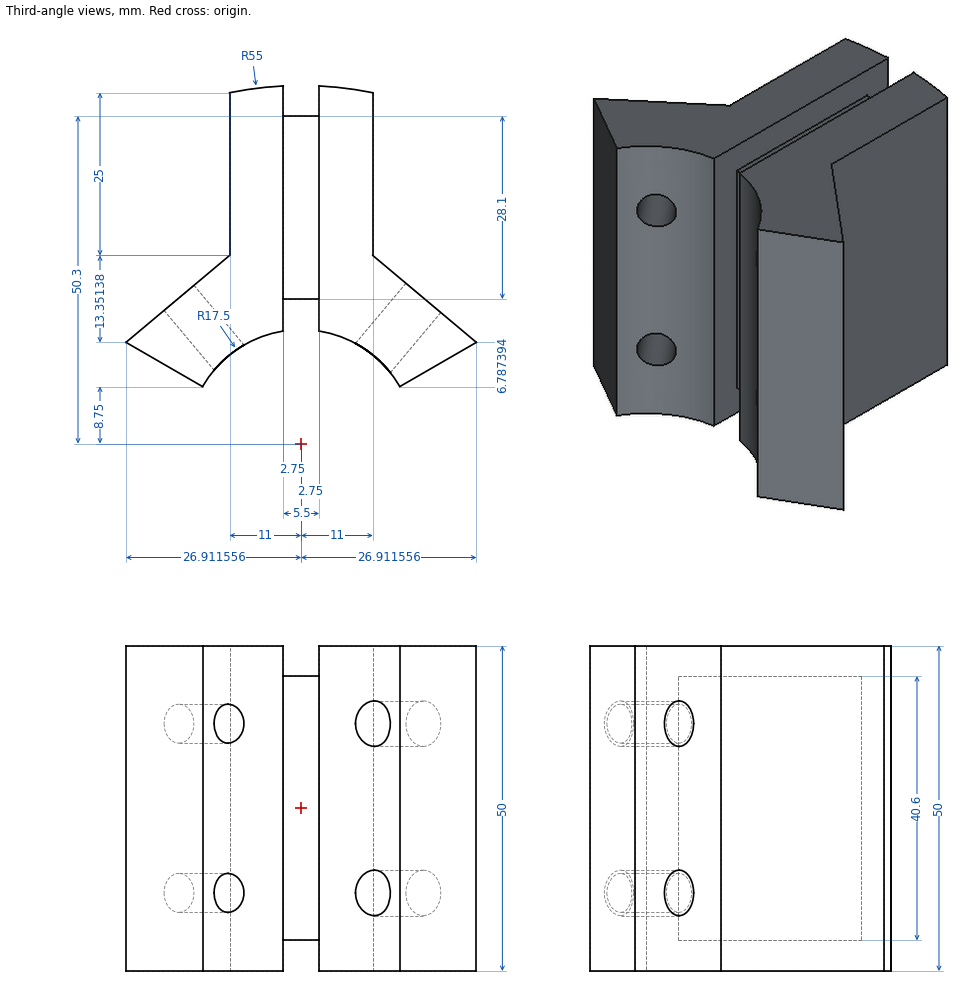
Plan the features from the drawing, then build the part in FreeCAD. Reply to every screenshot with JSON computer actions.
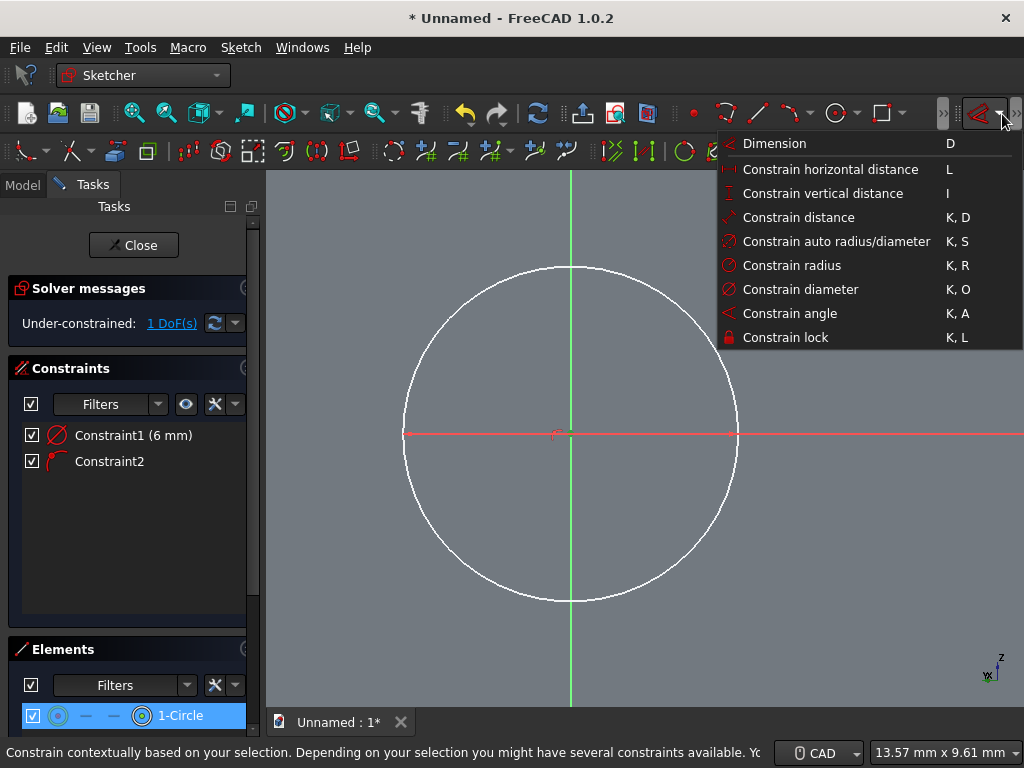
{"action": "left_click", "coordinate": [870, 193]}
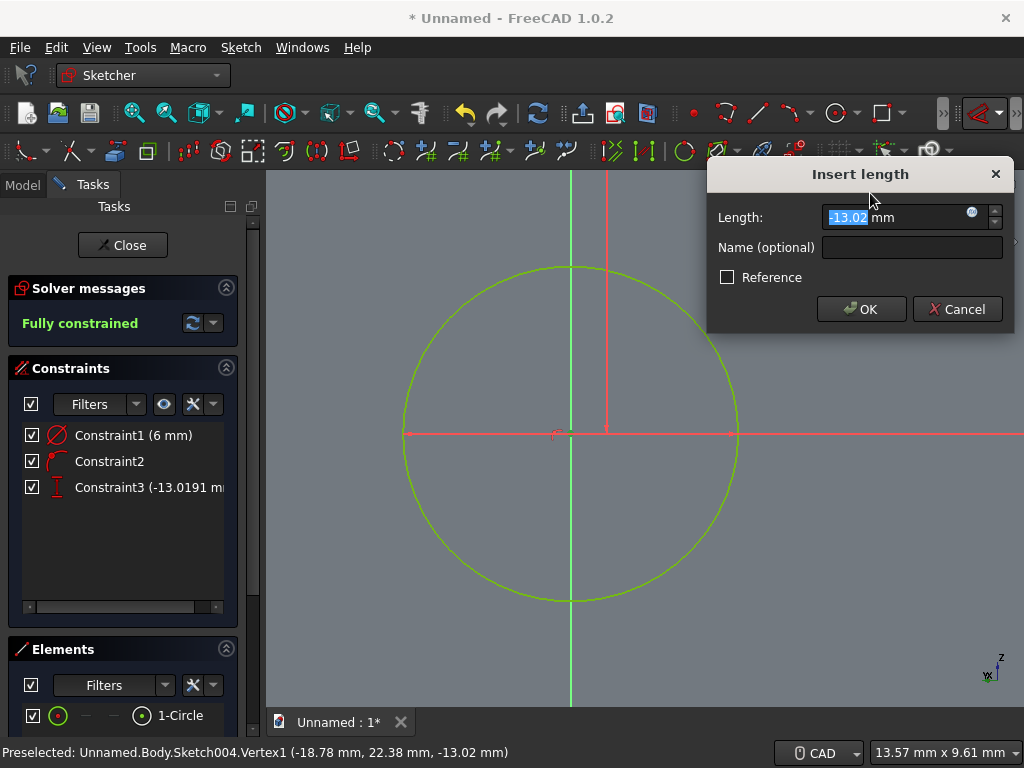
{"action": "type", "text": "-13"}
{"action": "key", "text": "Return"}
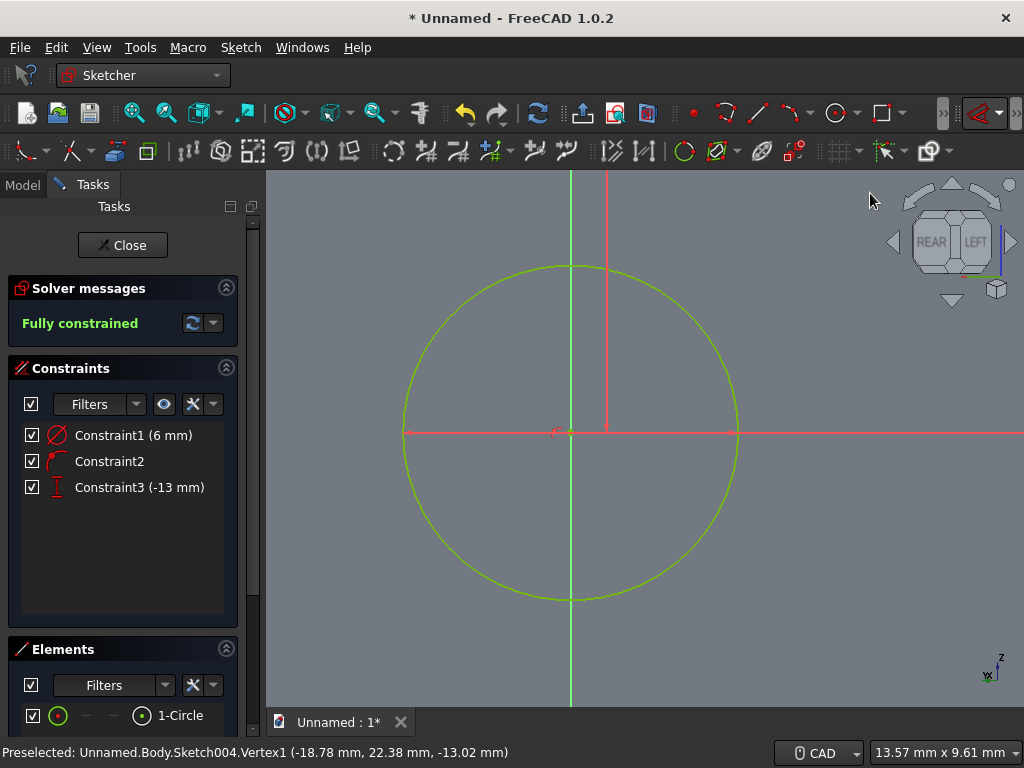
{"action": "left_click", "coordinate": [123, 245]}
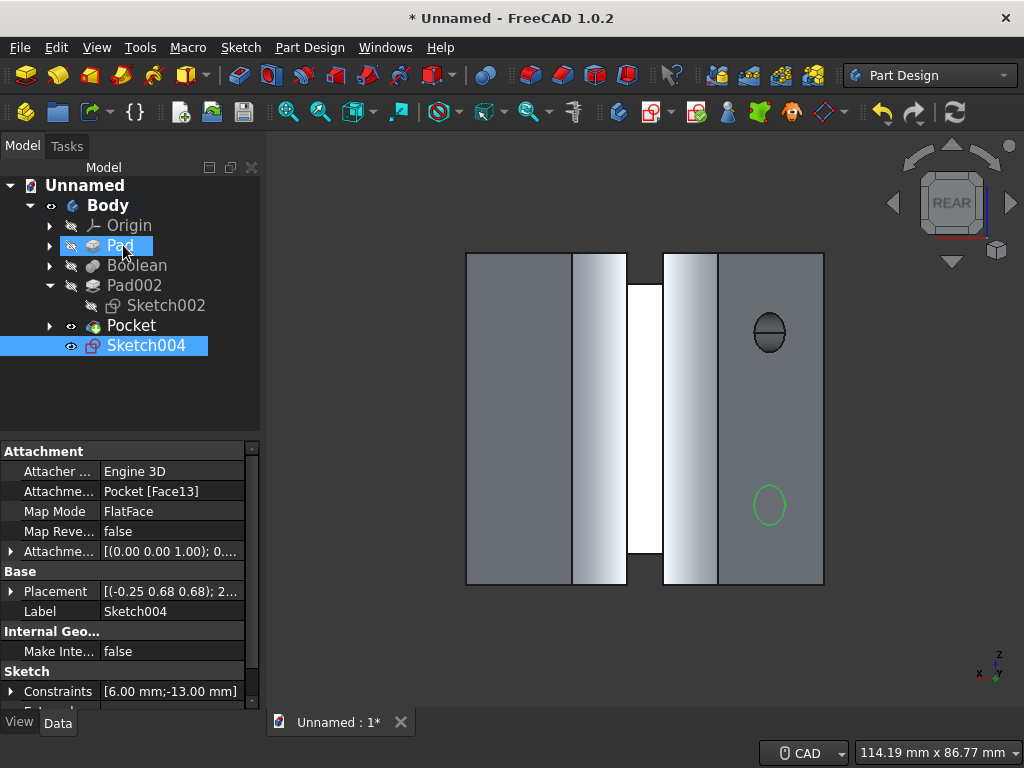
{"action": "left_click", "coordinate": [272, 76]}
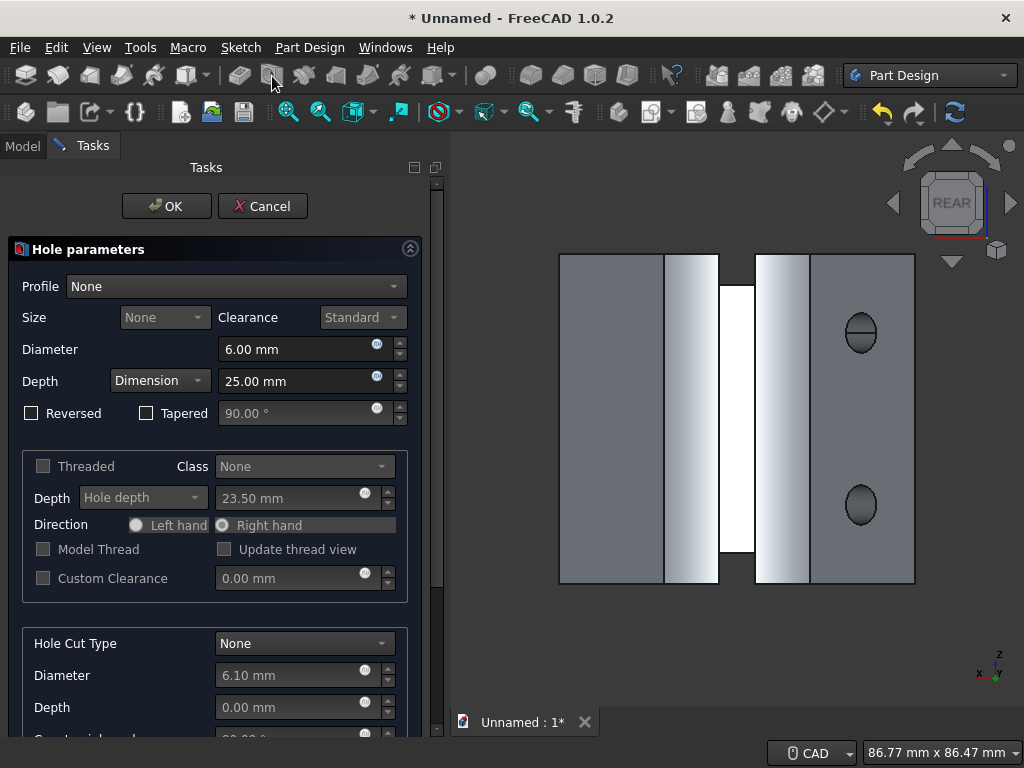
{"action": "triple_click", "coordinate": [305, 349]}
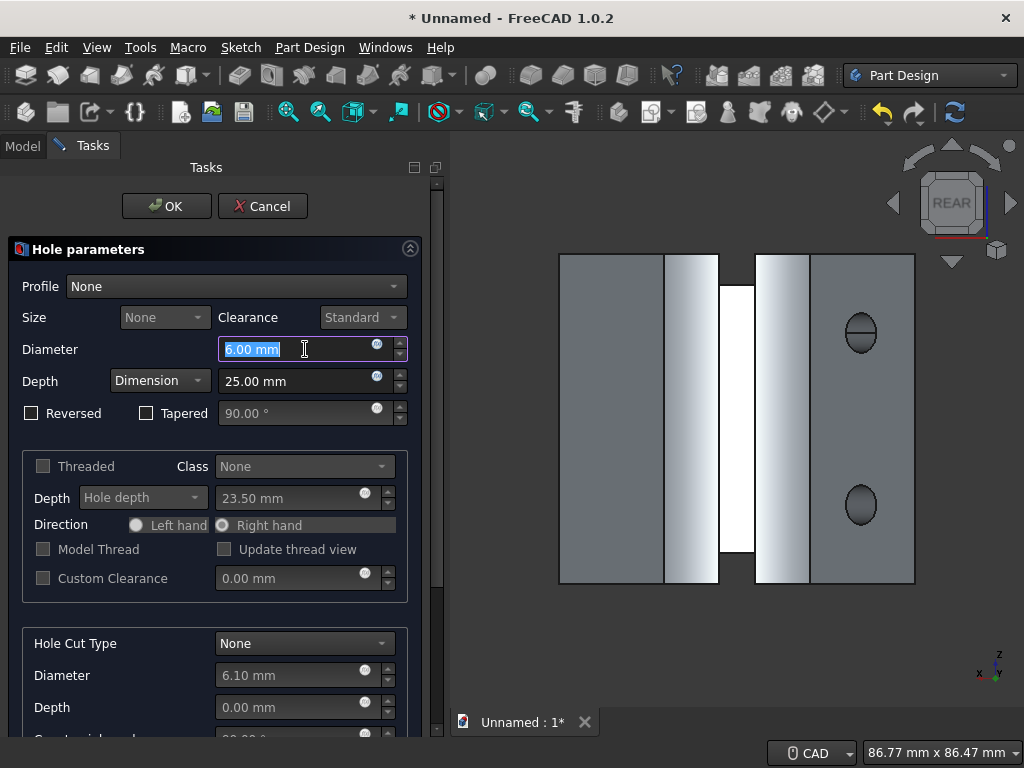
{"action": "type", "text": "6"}
{"action": "key", "text": "Tab"}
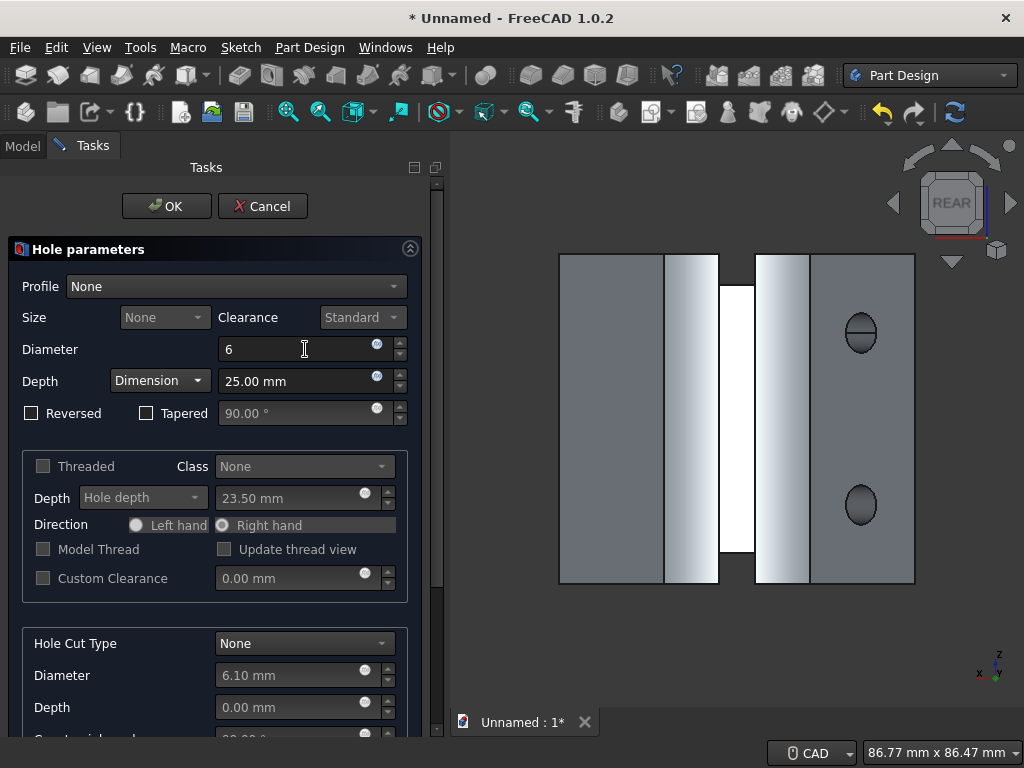
{"action": "left_click", "coordinate": [161, 380]}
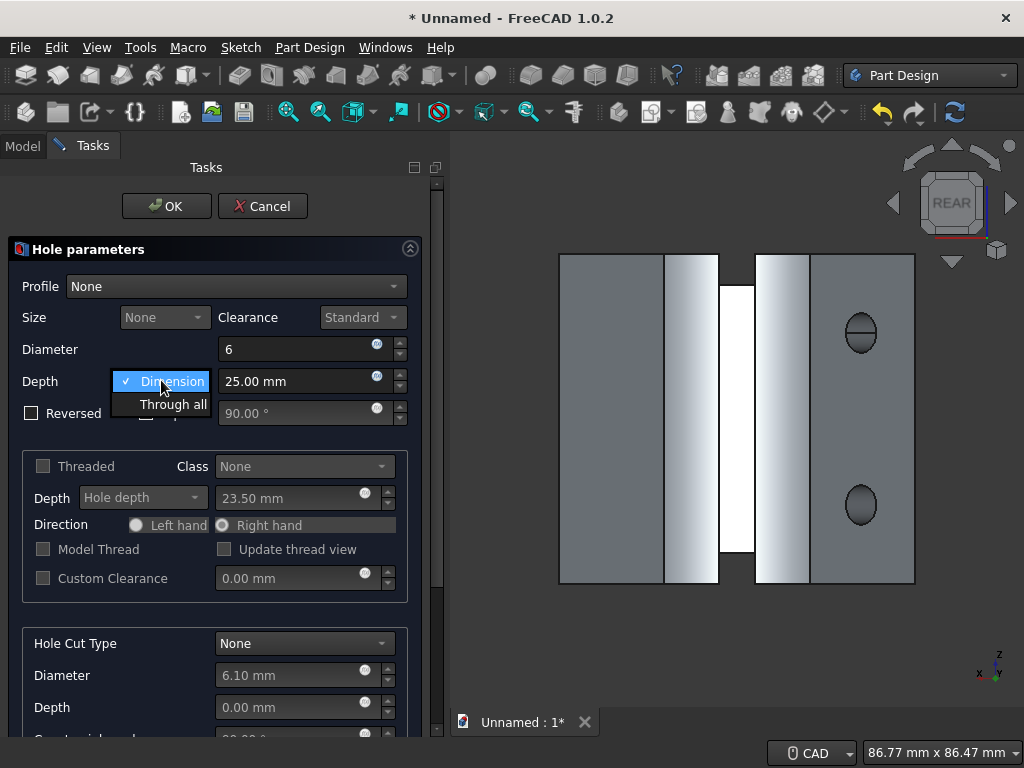
{"action": "left_click", "coordinate": [160, 404]}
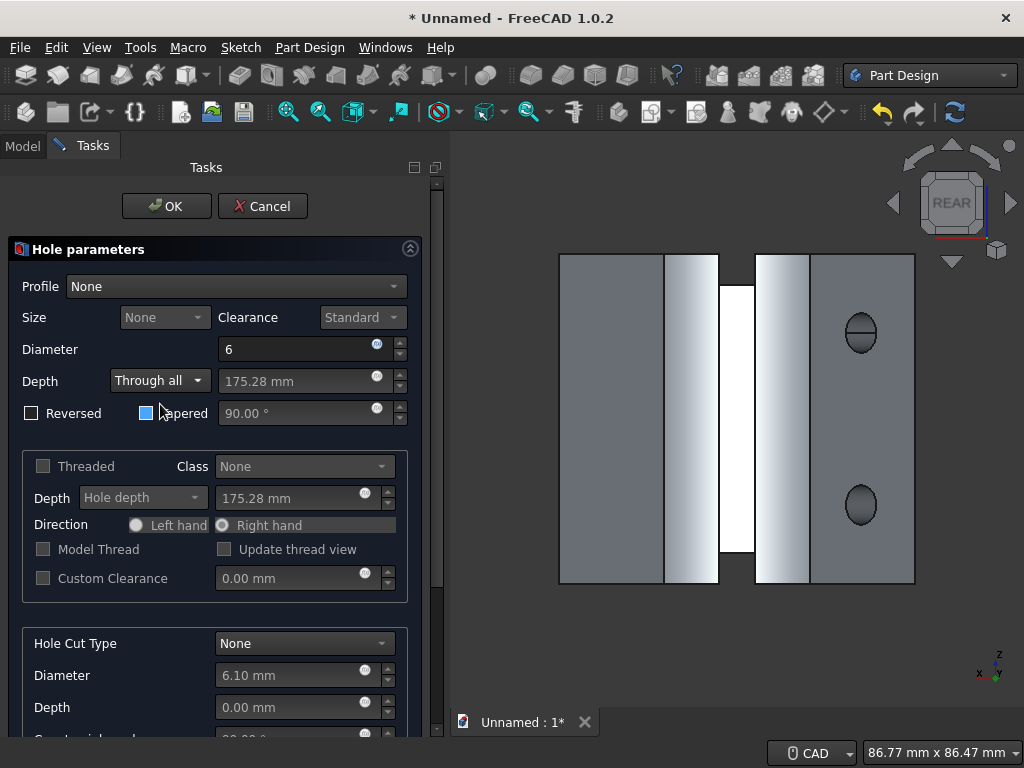
{"action": "left_click", "coordinate": [167, 206]}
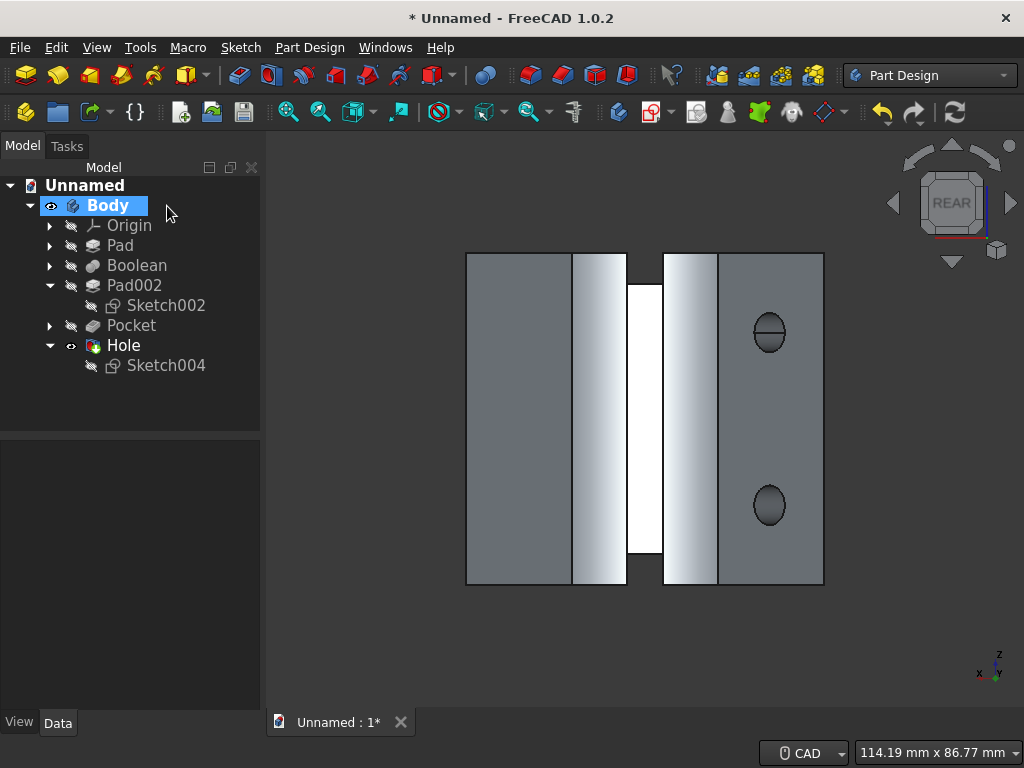
{"action": "left_click", "coordinate": [519, 323]}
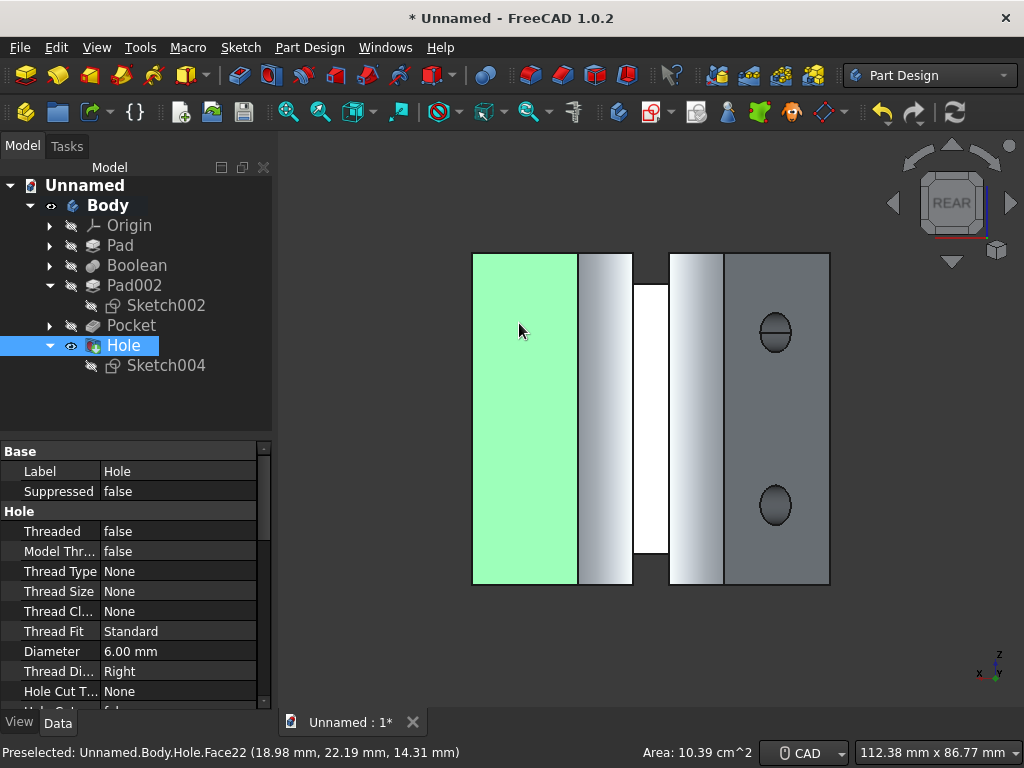
{"action": "left_click", "coordinate": [652, 112]}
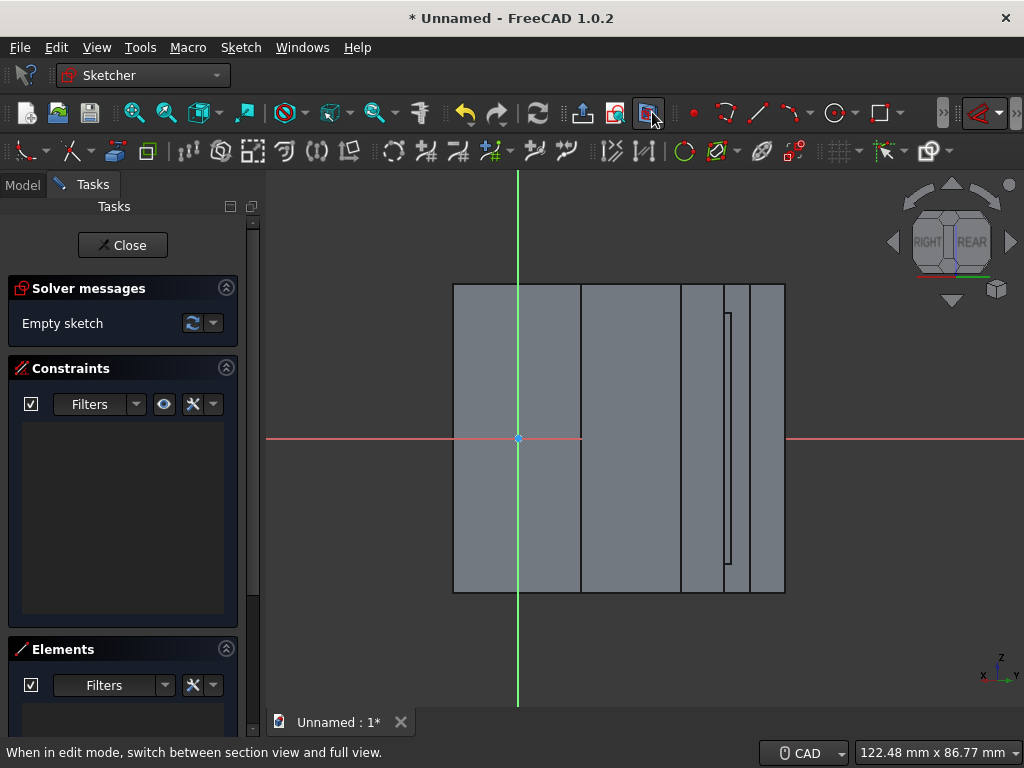
{"action": "scroll", "coordinate": [493, 365], "scroll_direction": "up", "scroll_amount": 6}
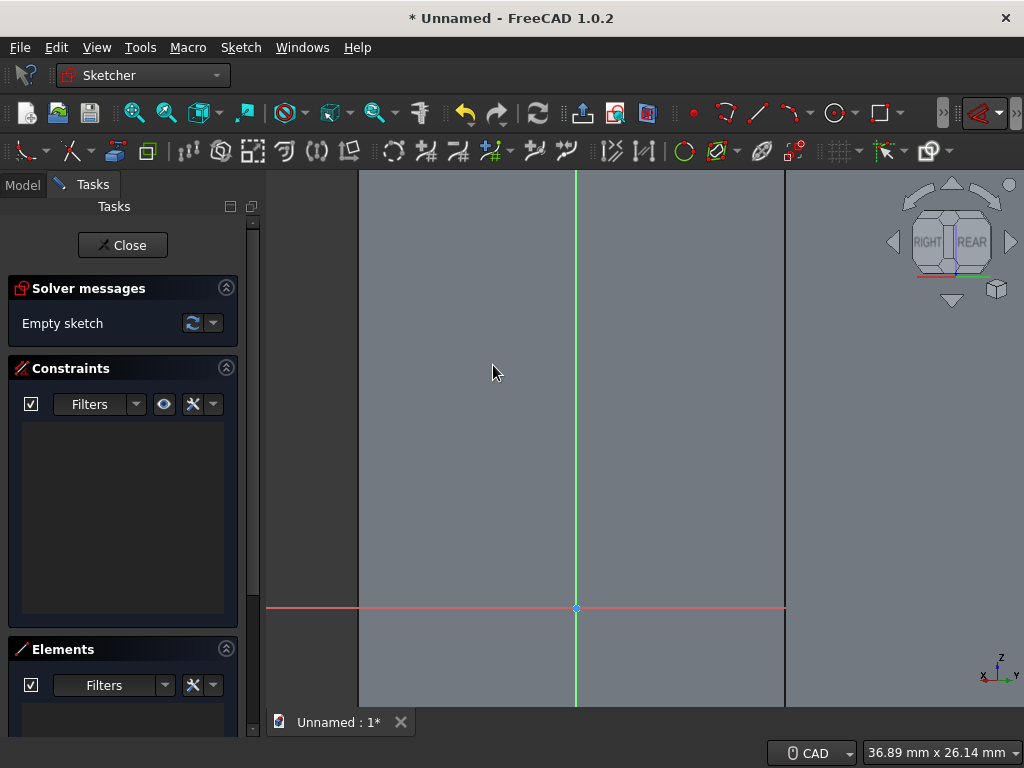
{"action": "left_click", "coordinate": [836, 114]}